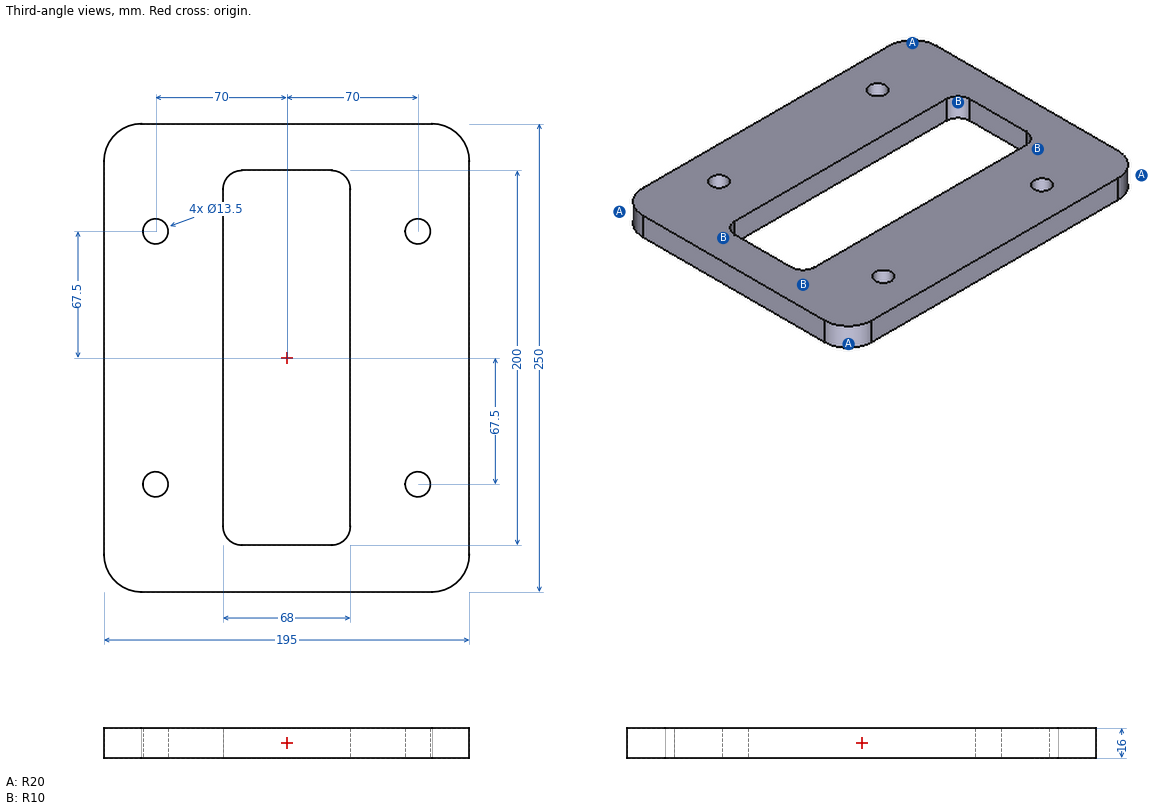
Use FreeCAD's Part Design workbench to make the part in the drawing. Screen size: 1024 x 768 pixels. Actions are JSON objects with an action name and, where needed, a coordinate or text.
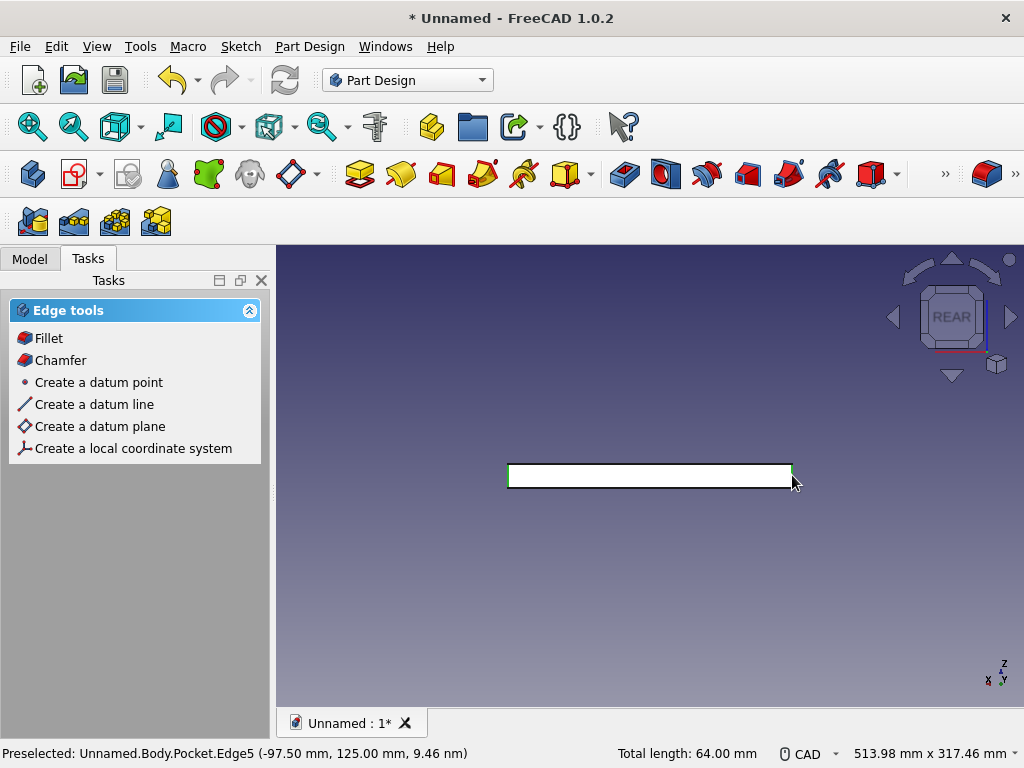
{"action": "left_click", "coordinate": [987, 174]}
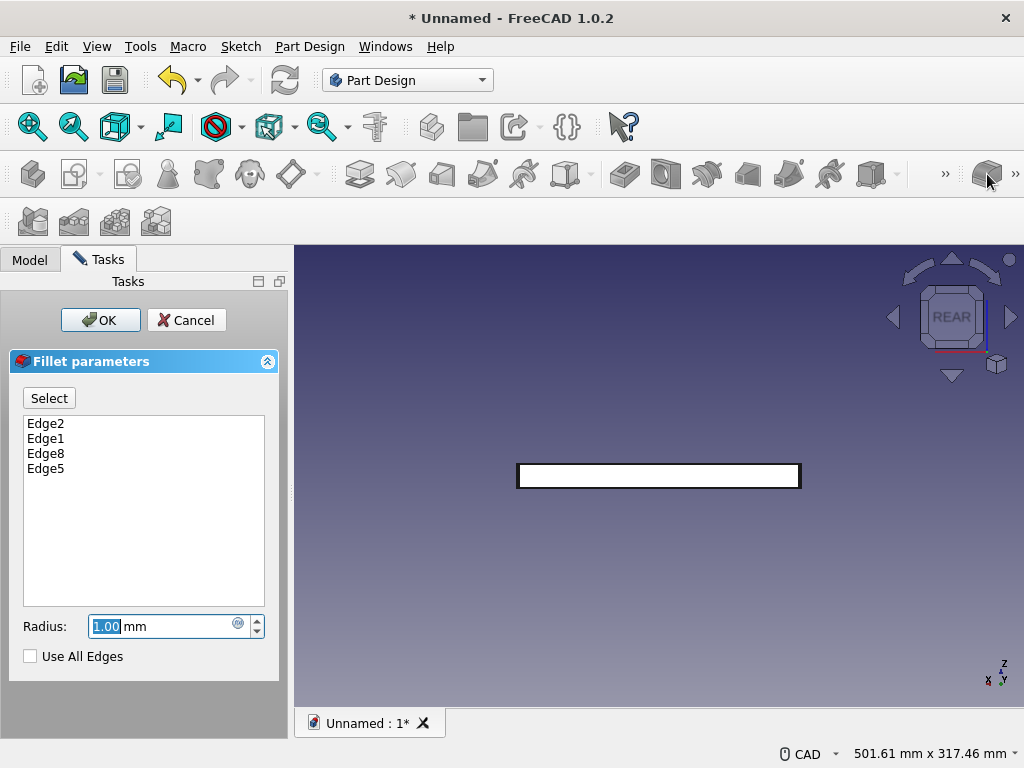
{"action": "type", "text": "20"}
{"action": "key", "text": "Tab"}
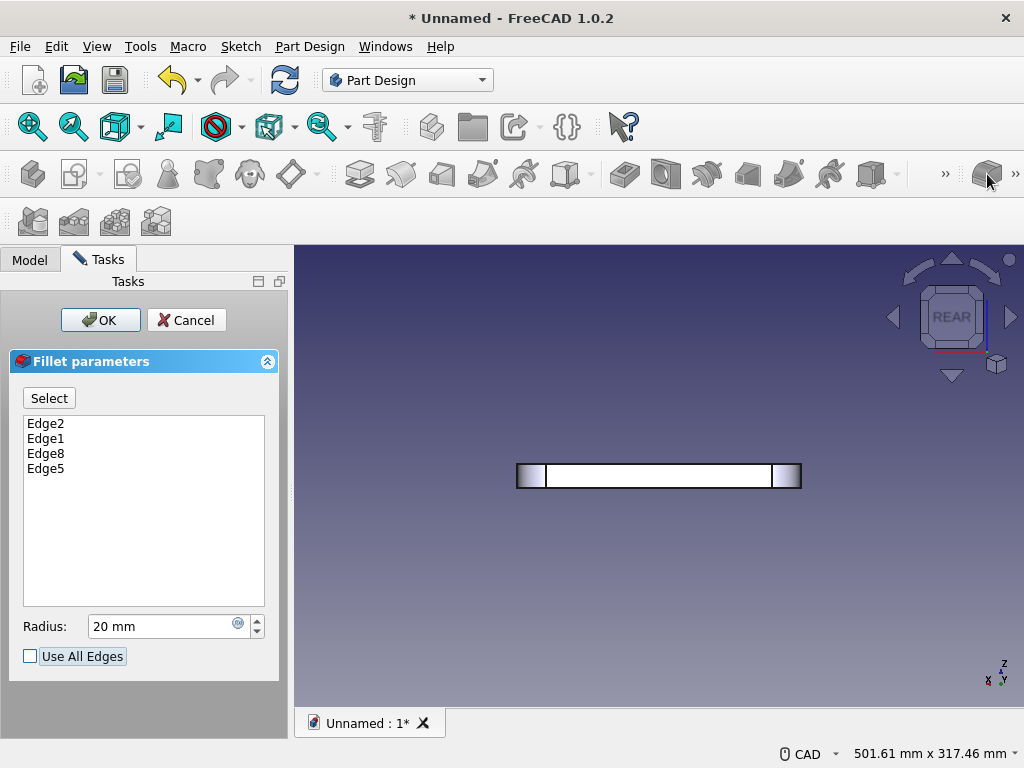
{"action": "left_click", "coordinate": [101, 320]}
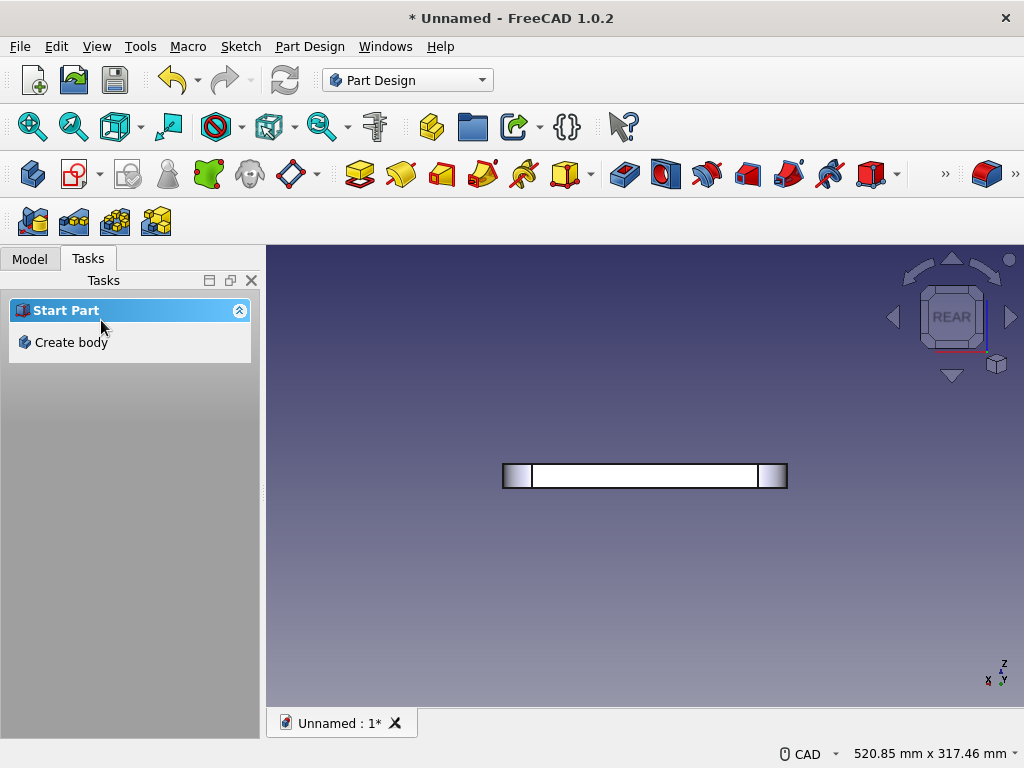
{"action": "left_click", "coordinate": [33, 128]}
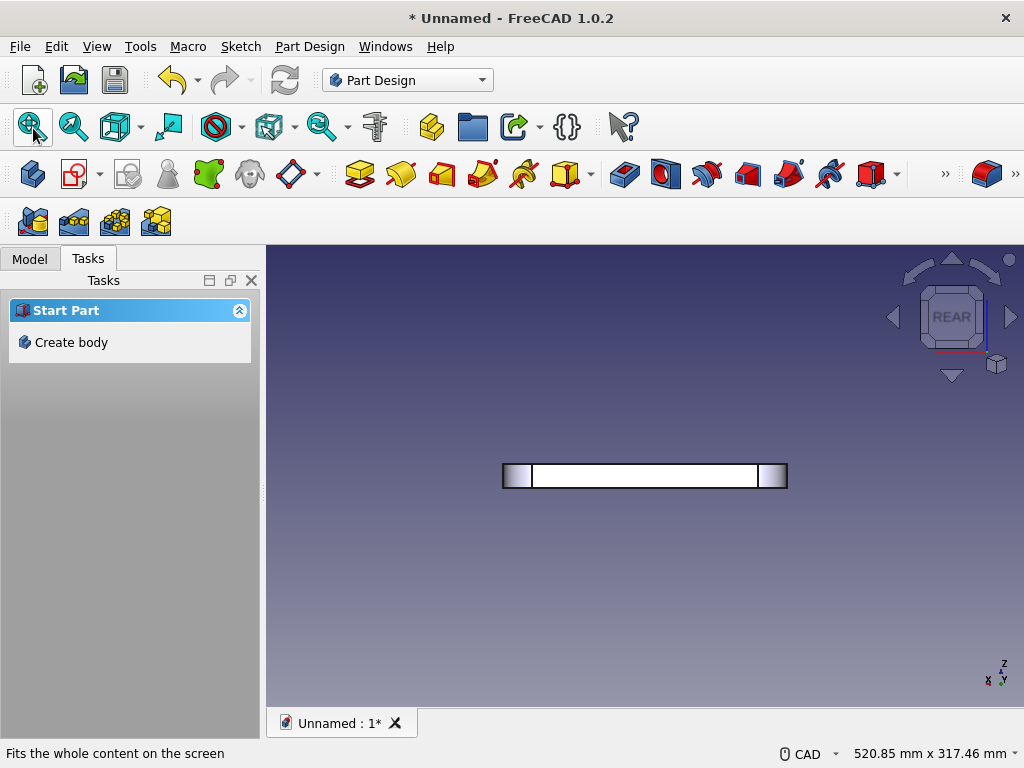
{"action": "key", "text": "0"}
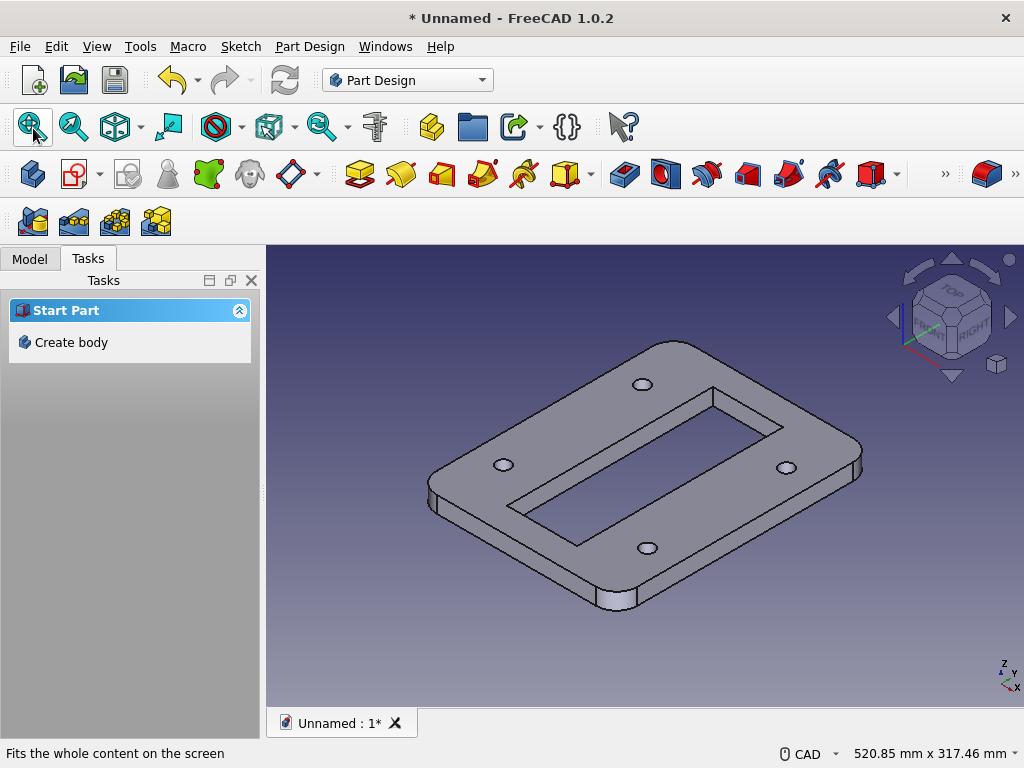
{"action": "key", "text": "2"}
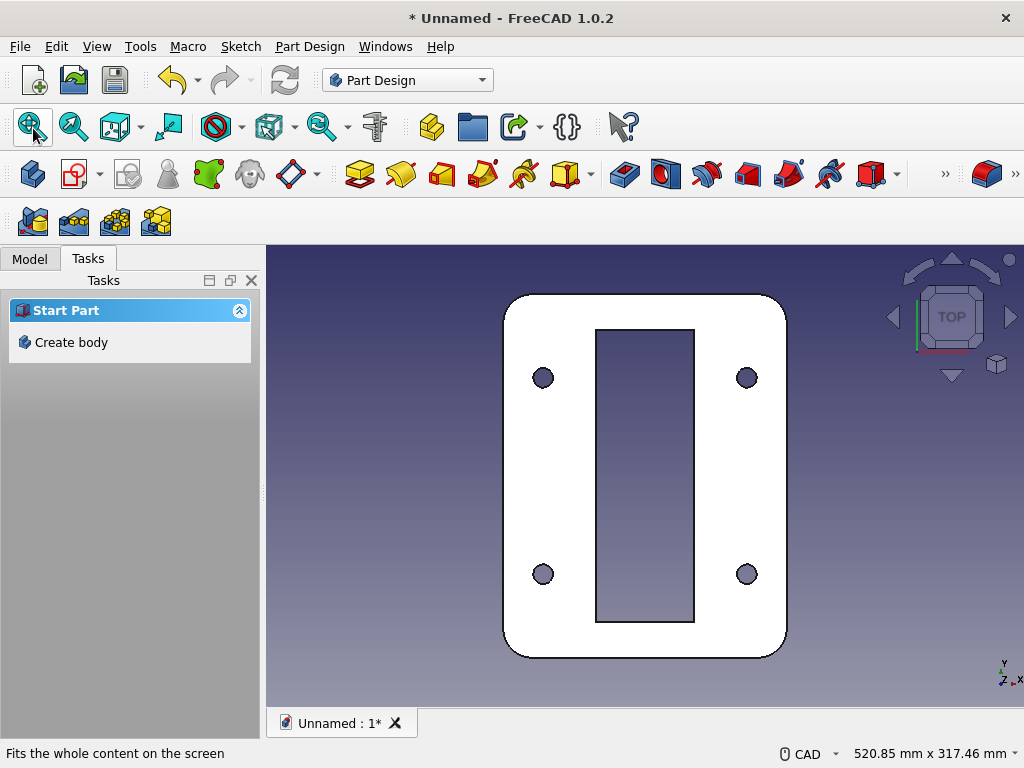
{"action": "key", "text": "1"}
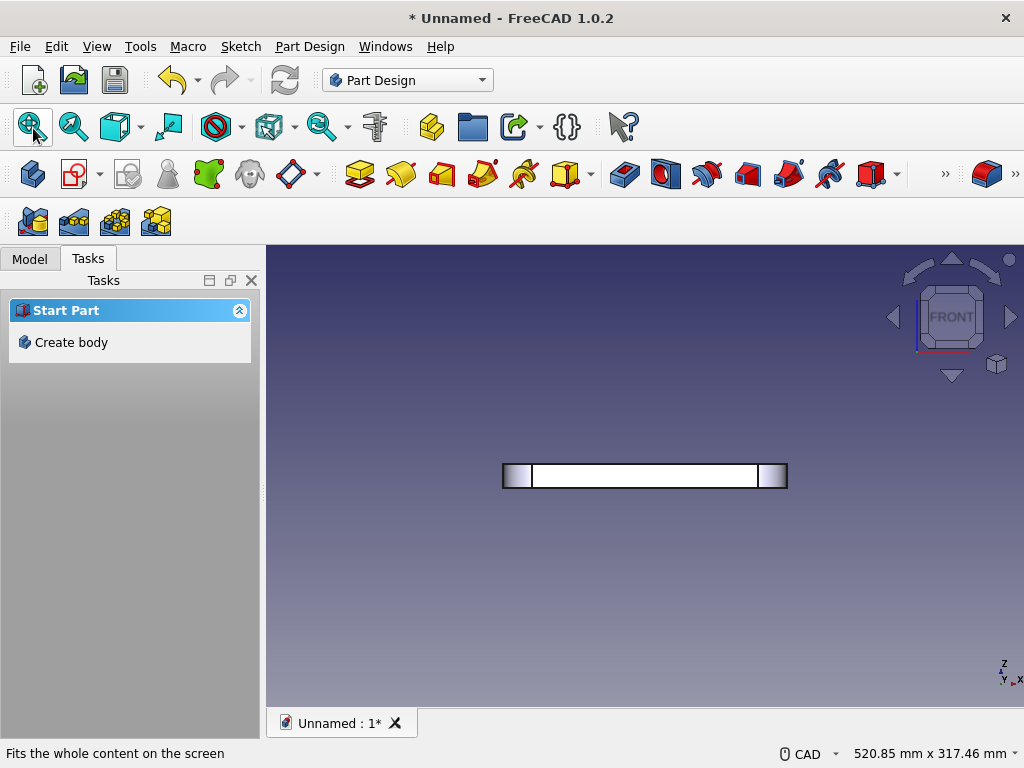
{"action": "left_click", "coordinate": [33, 128]}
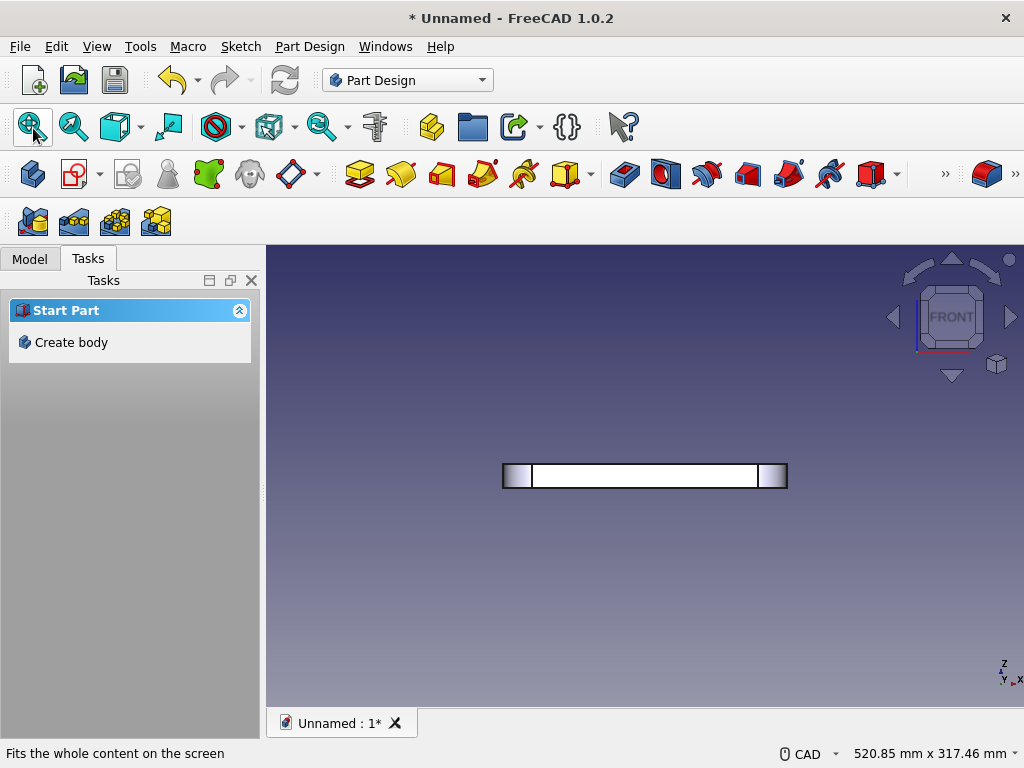
{"action": "key", "text": "3"}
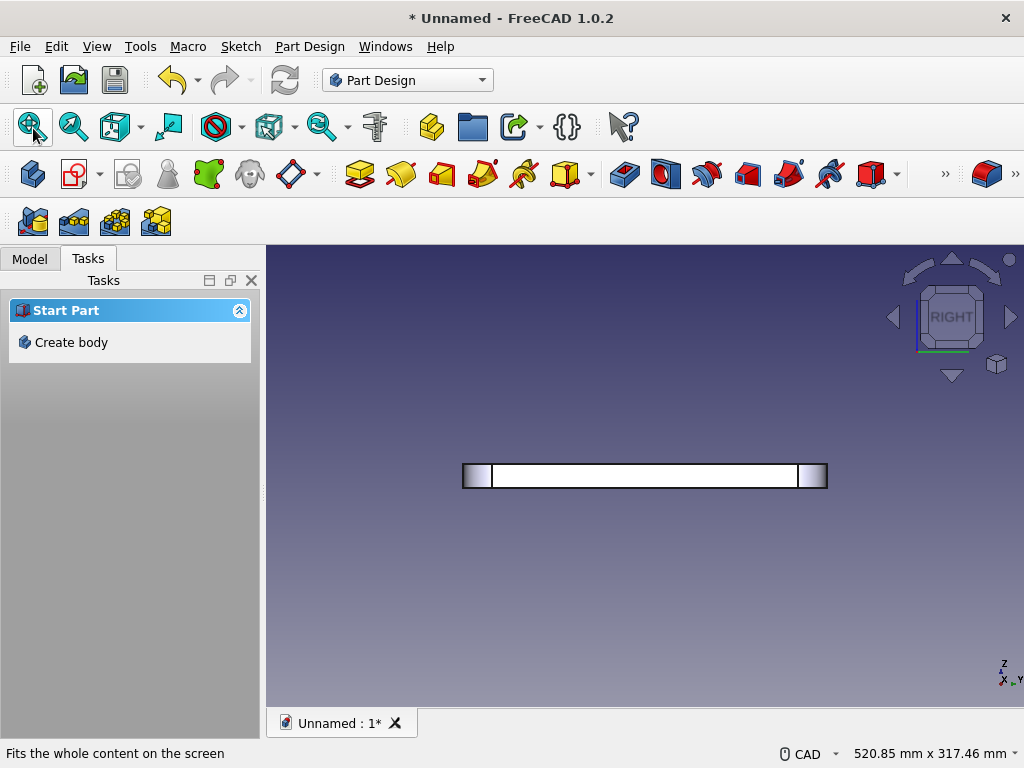
{"action": "key", "text": "5"}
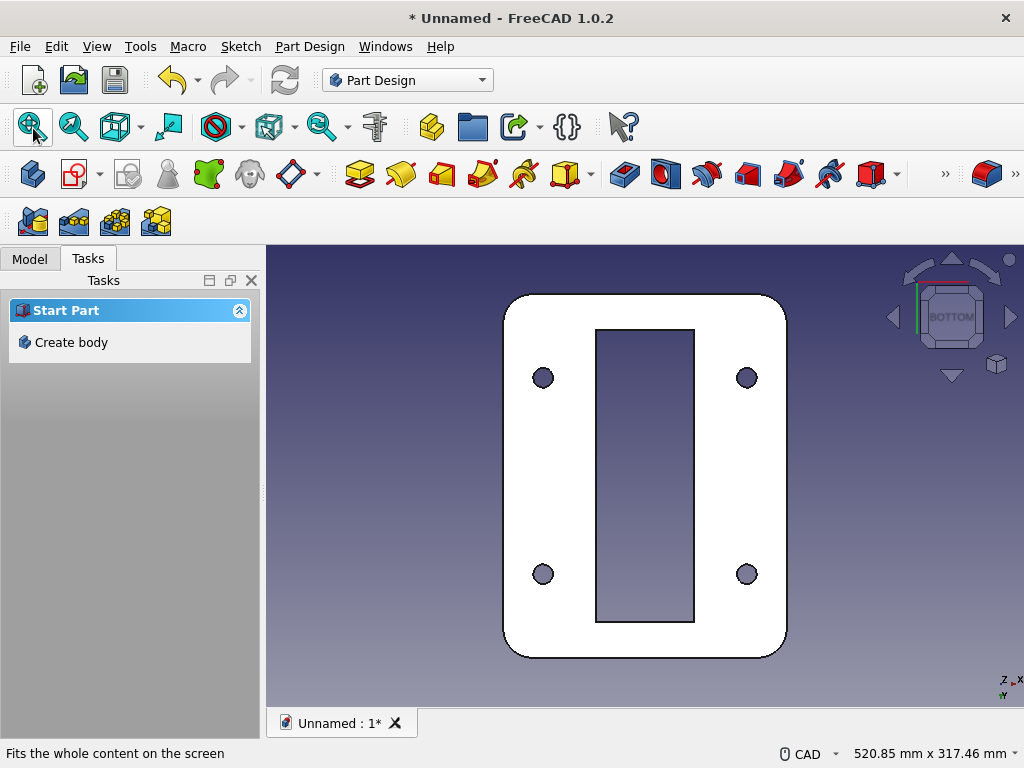
{"action": "key", "text": "4"}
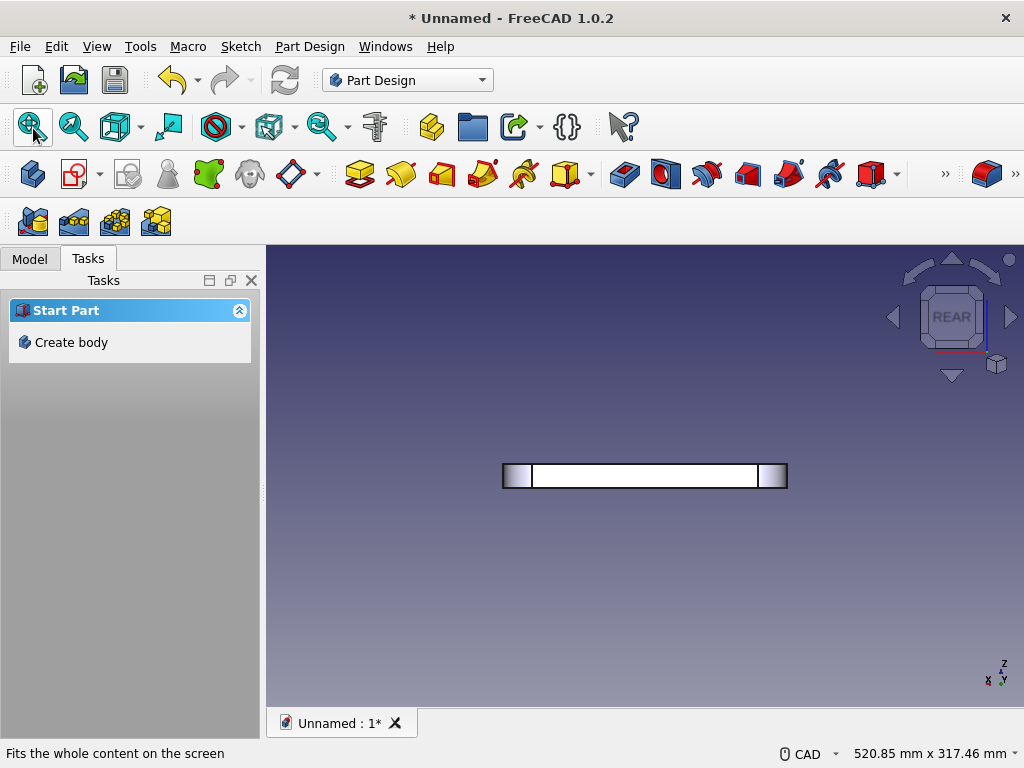
{"action": "left_click", "coordinate": [33, 128]}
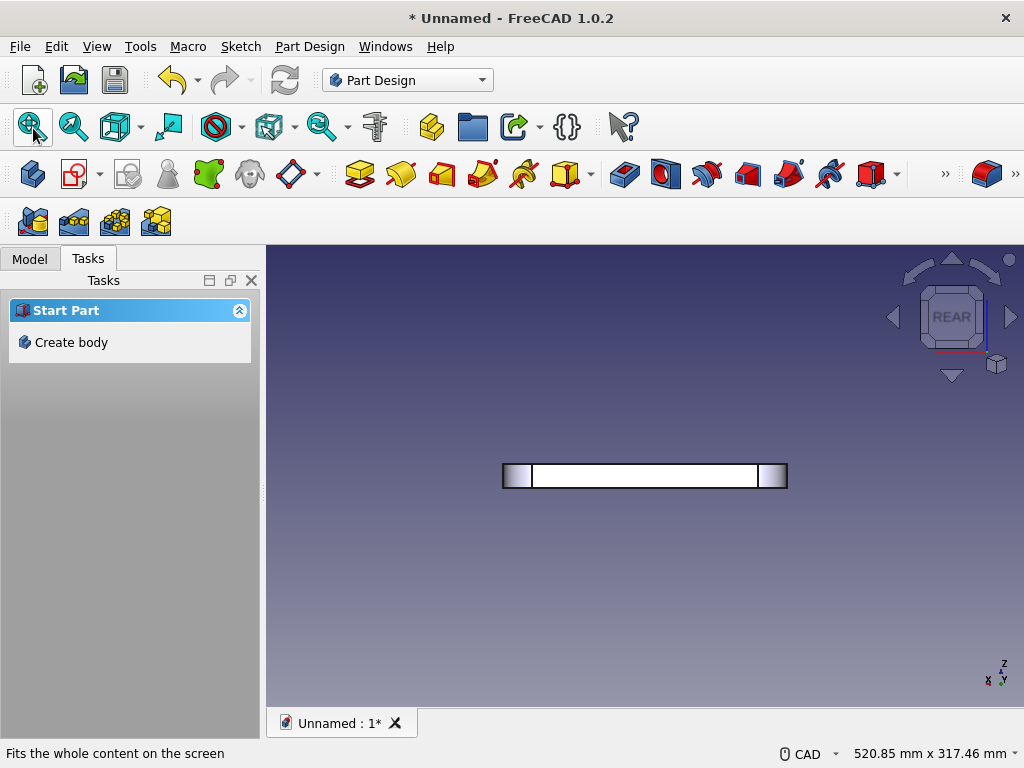
{"action": "key", "text": "6"}